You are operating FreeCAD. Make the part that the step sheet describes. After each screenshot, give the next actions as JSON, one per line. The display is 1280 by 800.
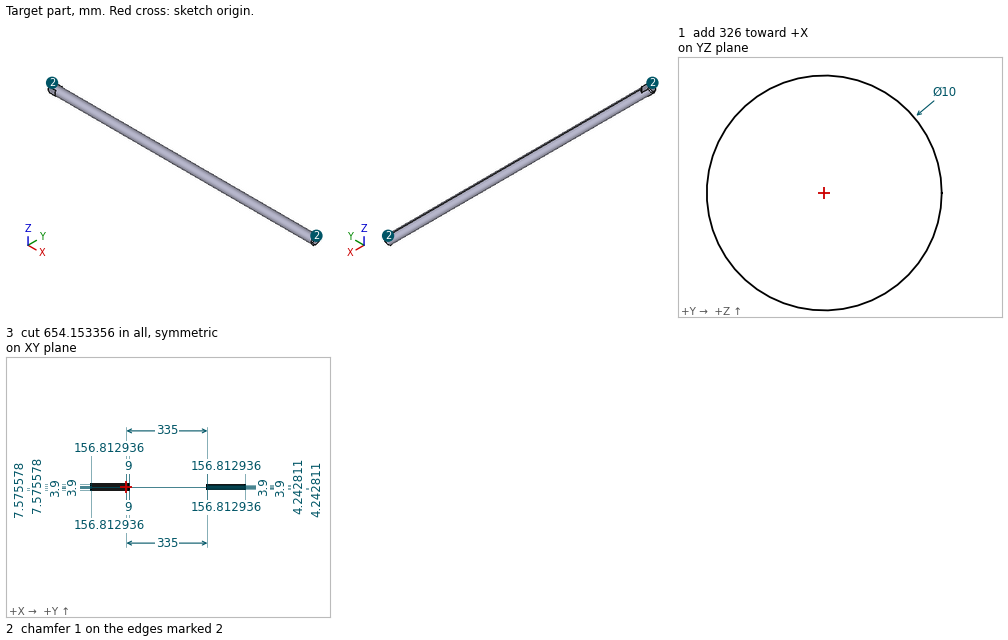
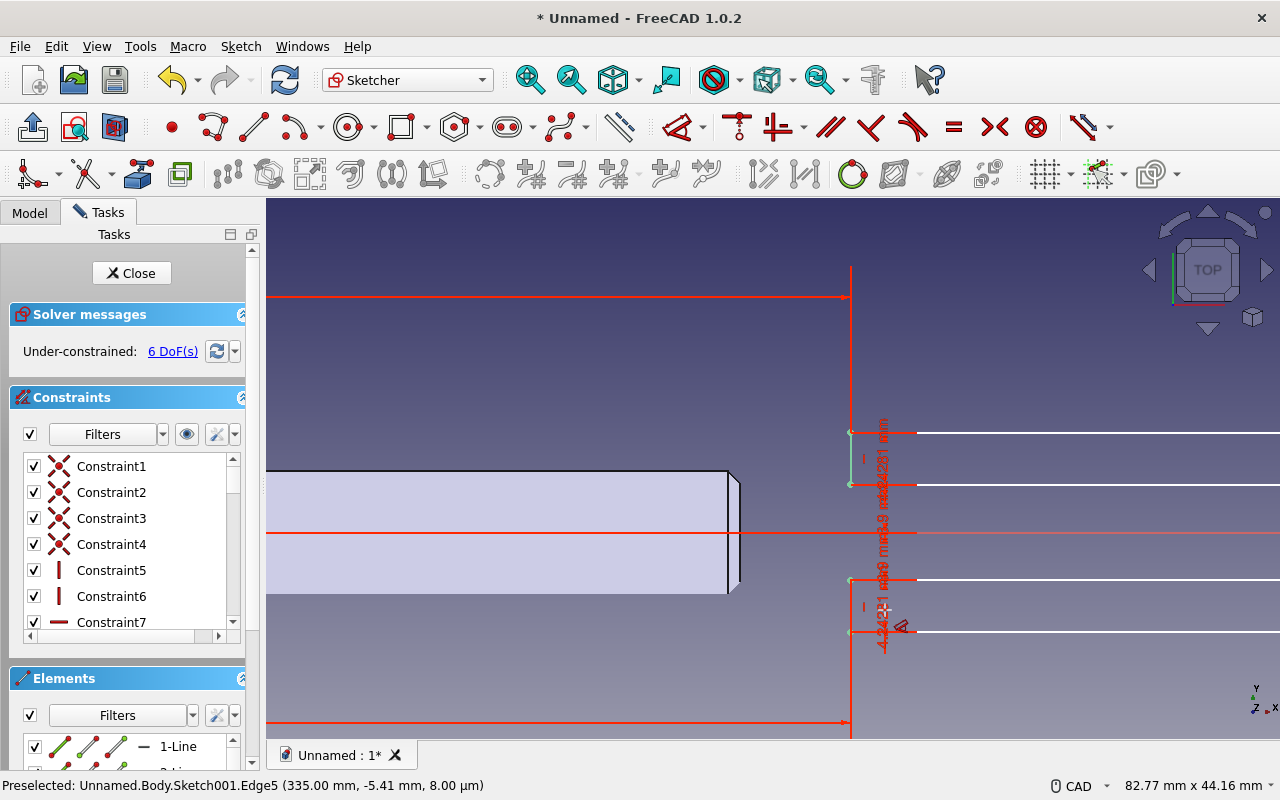
{"action": "scroll", "coordinate": [853, 463], "scroll_direction": "down", "scroll_amount": 13}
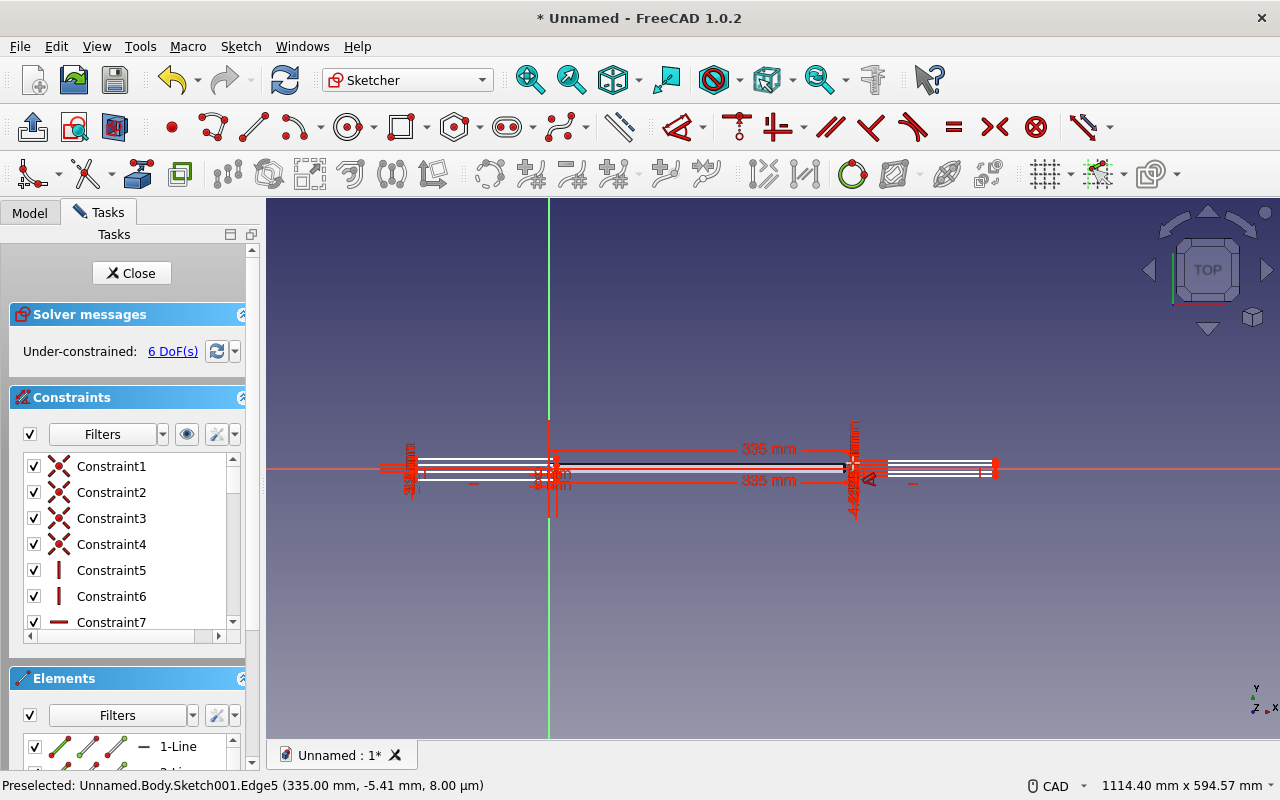
{"action": "scroll", "coordinate": [414, 461], "scroll_direction": "up", "scroll_amount": 10}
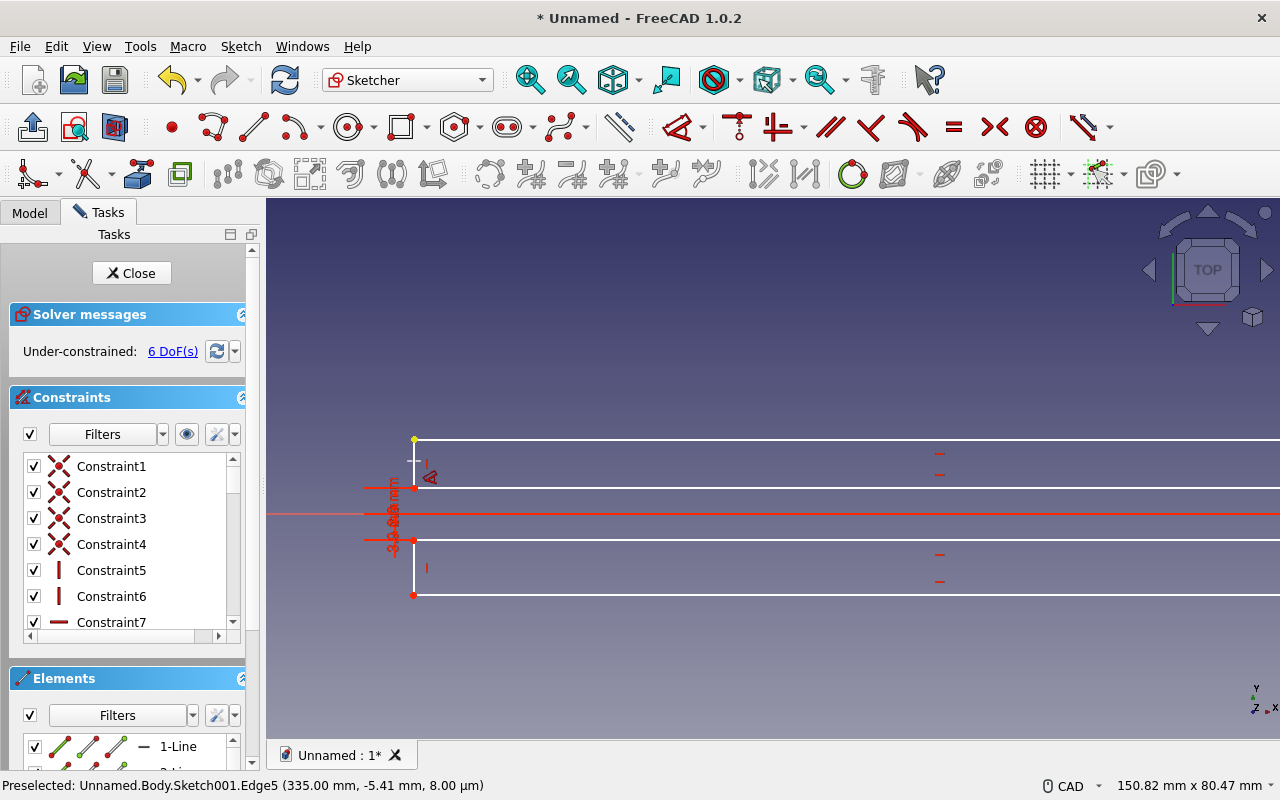
{"action": "left_click", "coordinate": [414, 454]}
{"action": "left_click", "coordinate": [380, 464]}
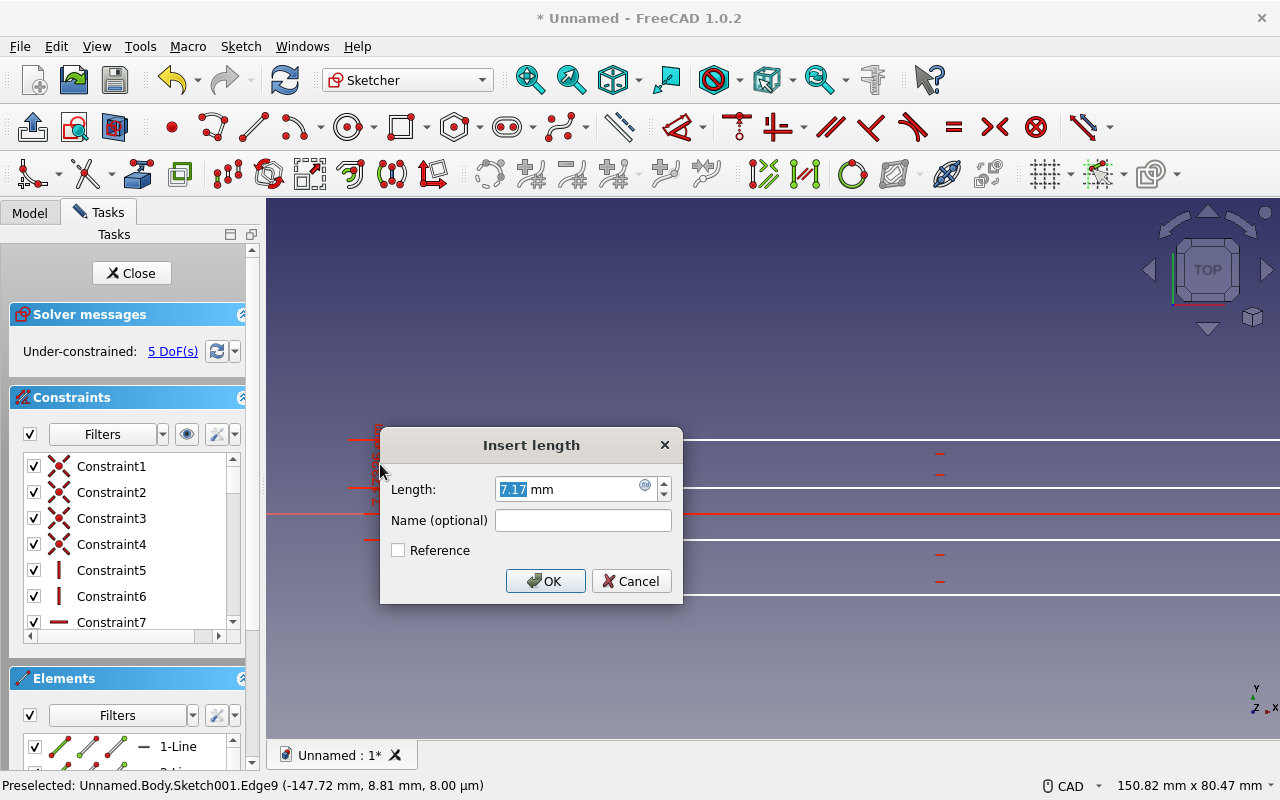
{"action": "type", "text": "7.575578"}
{"action": "key", "text": "Return"}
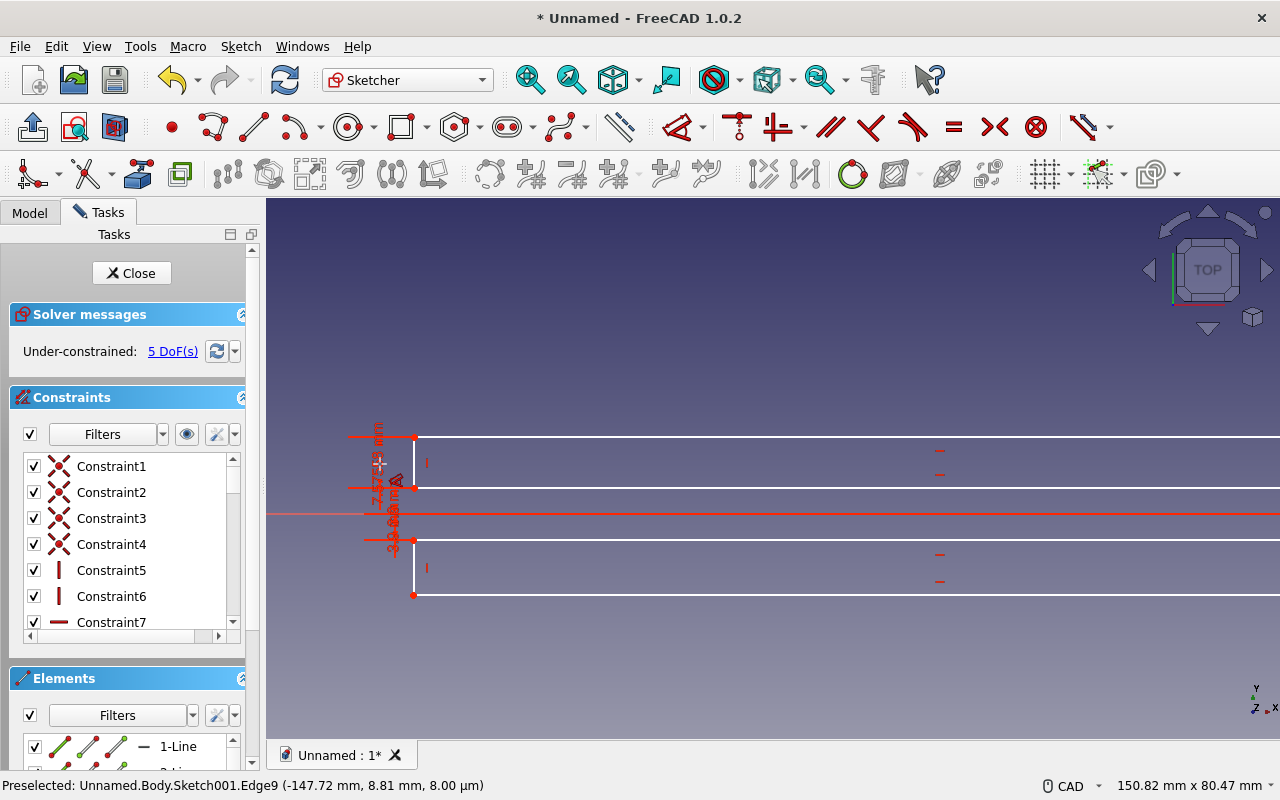
{"action": "left_click", "coordinate": [414, 557]}
{"action": "left_click", "coordinate": [380, 568]}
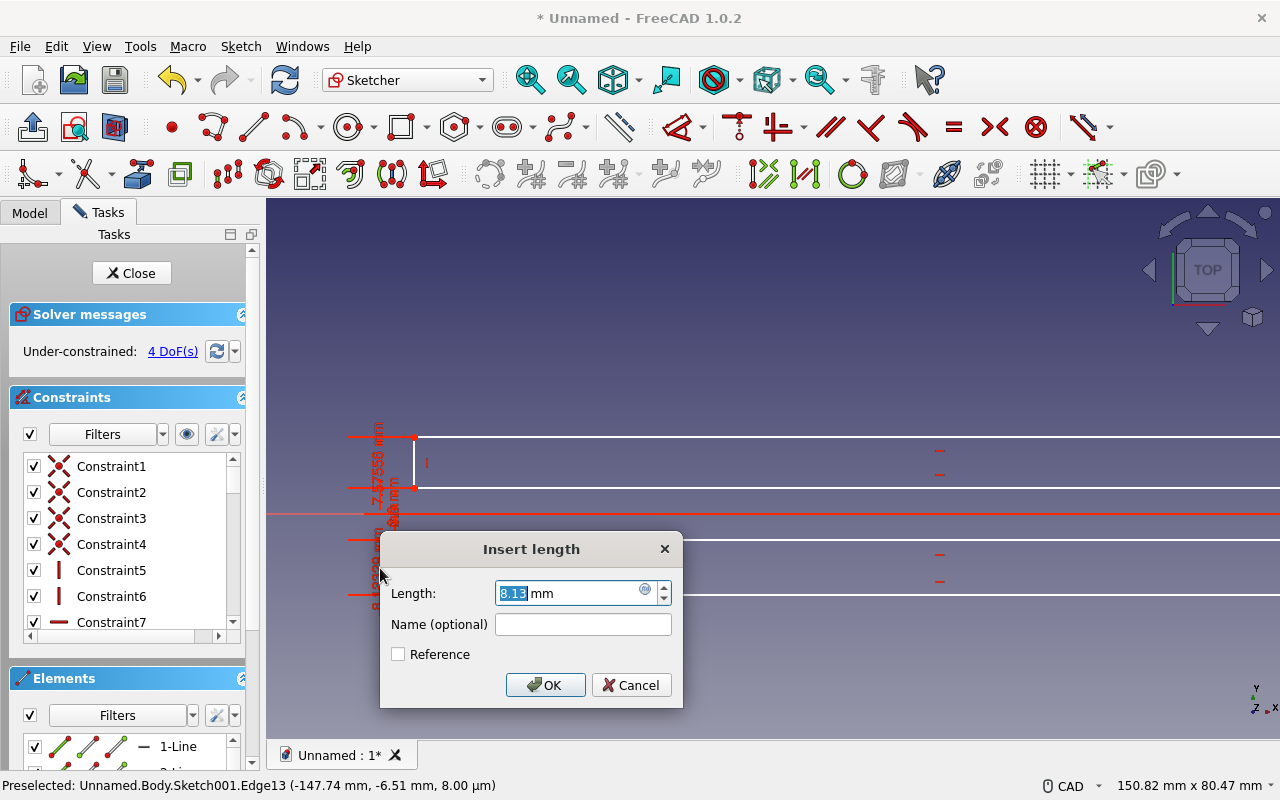
{"action": "type", "text": "7.575578"}
{"action": "key", "text": "Return"}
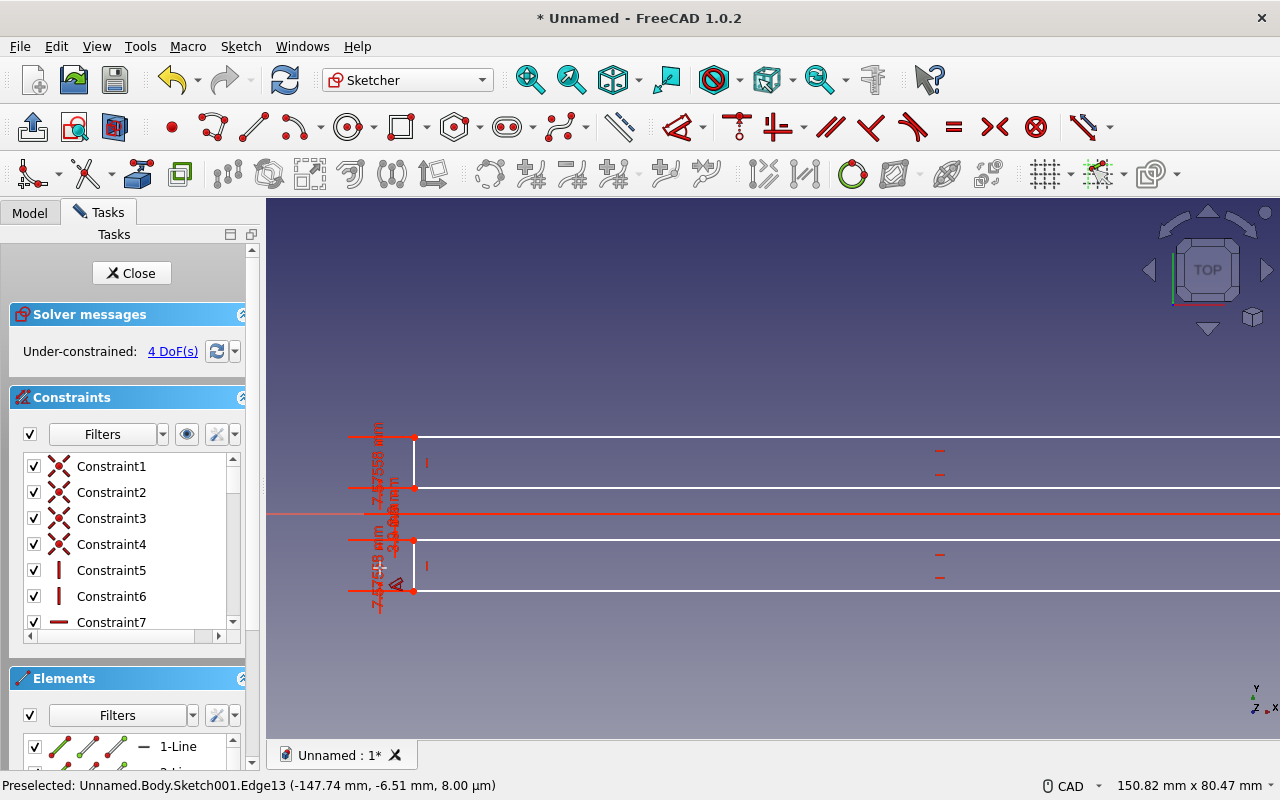
{"action": "scroll", "coordinate": [414, 461], "scroll_direction": "down", "scroll_amount": 10}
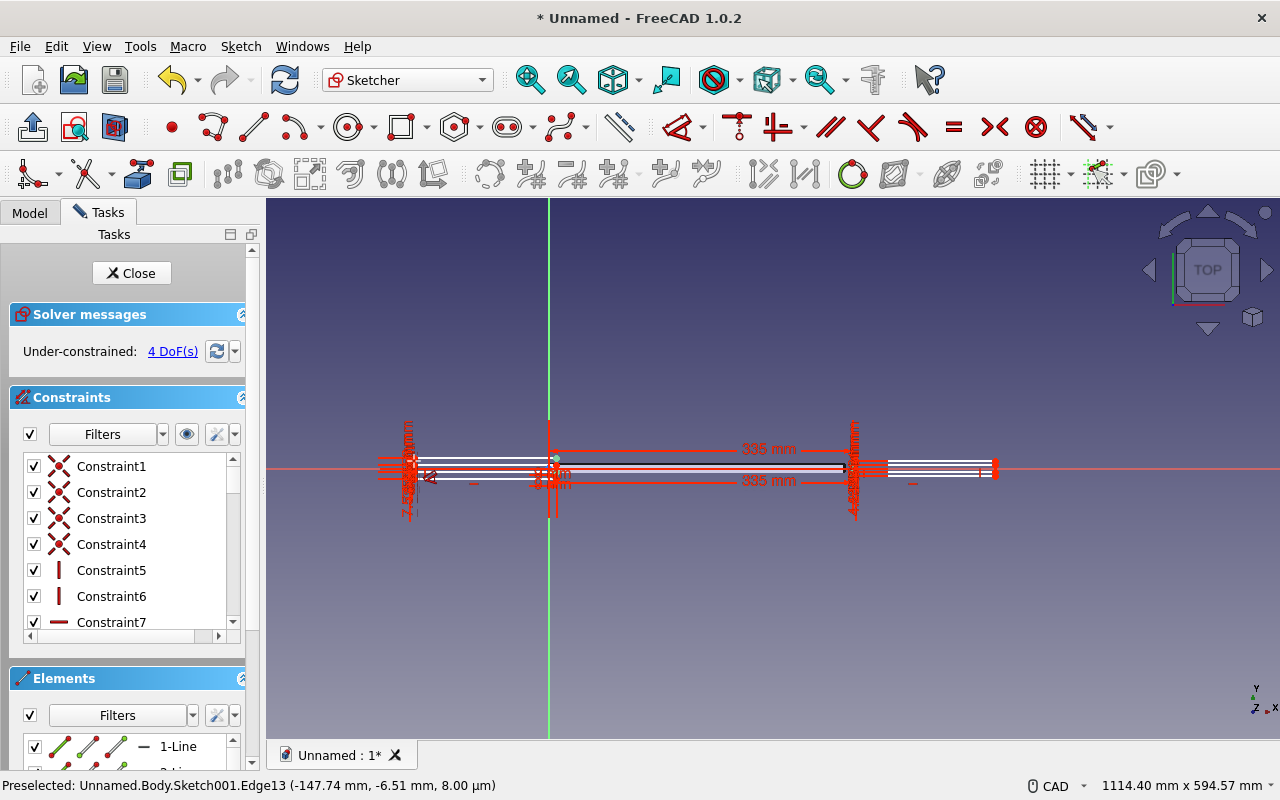
{"action": "scroll", "coordinate": [896, 465], "scroll_direction": "up", "scroll_amount": 7}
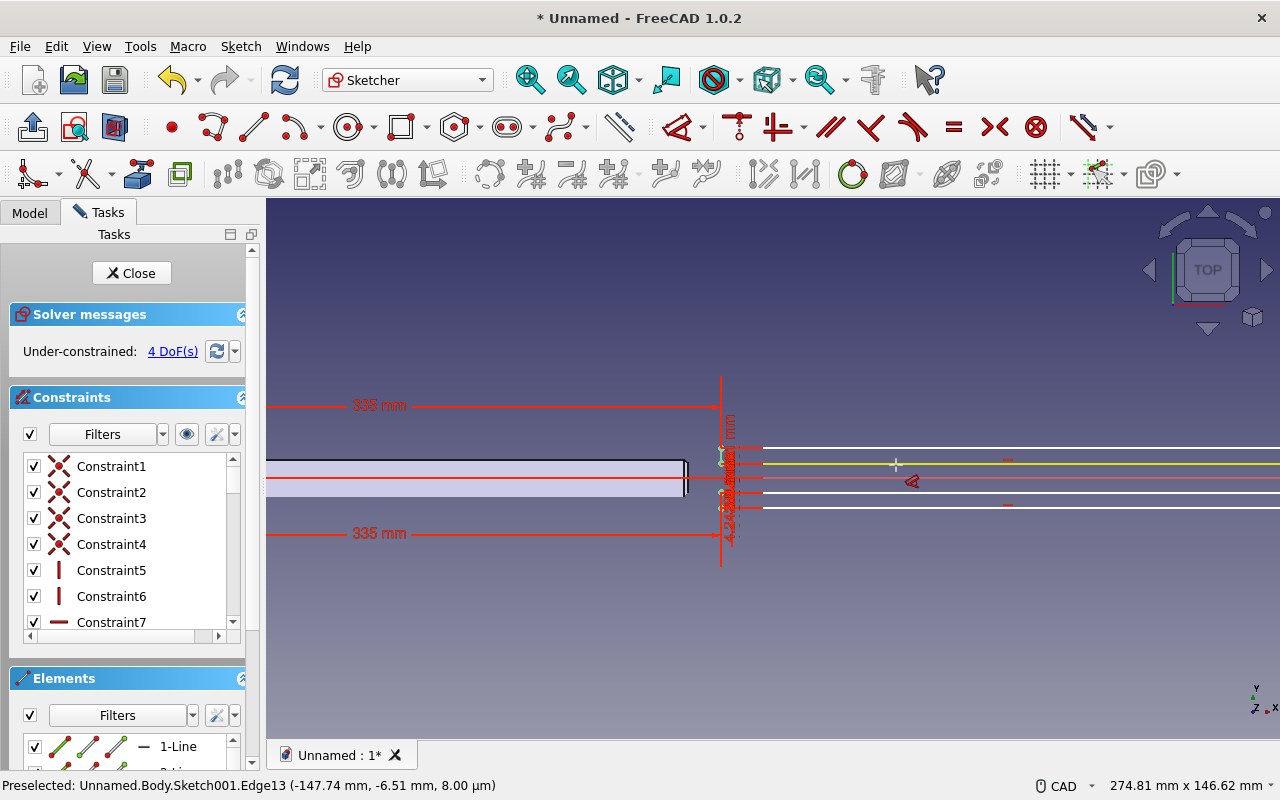
{"action": "left_click", "coordinate": [895, 464]}
{"action": "left_click", "coordinate": [918, 430]}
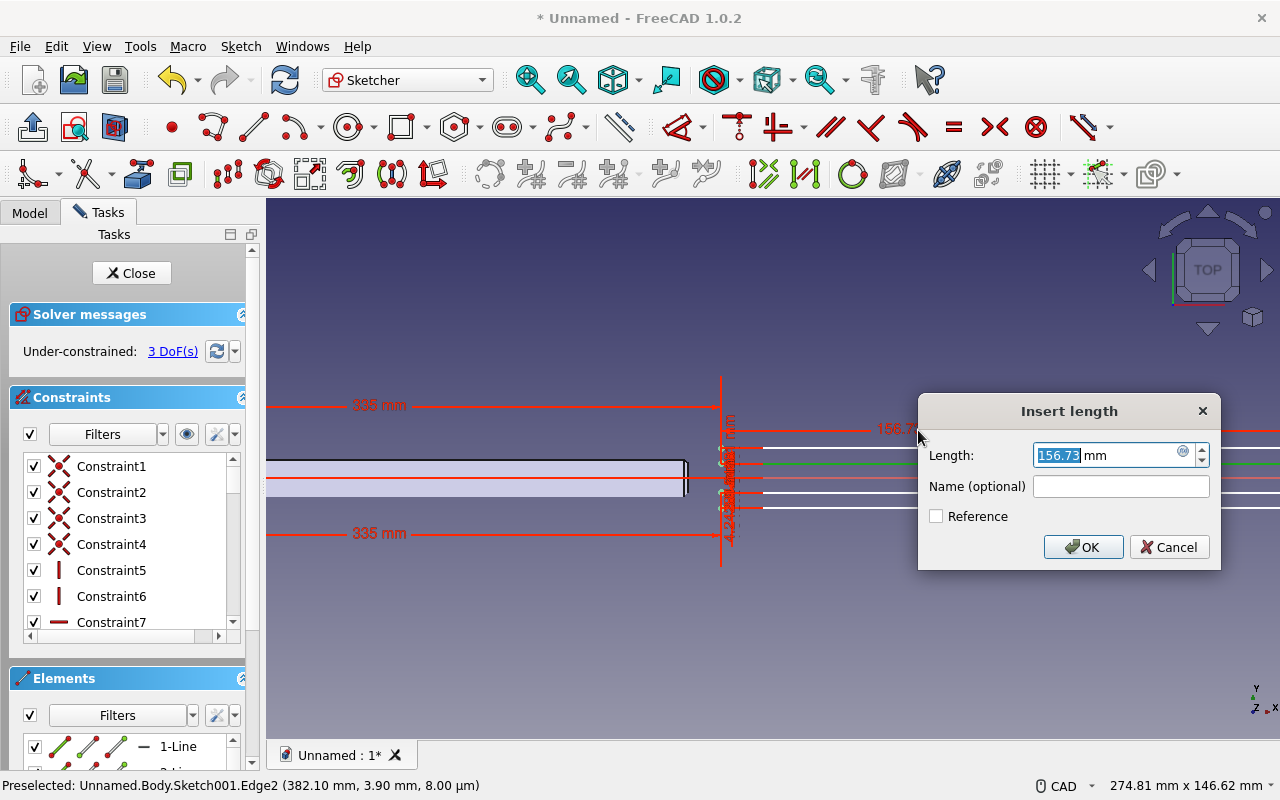
{"action": "type", "text": "156.812936"}
{"action": "key", "text": "Return"}